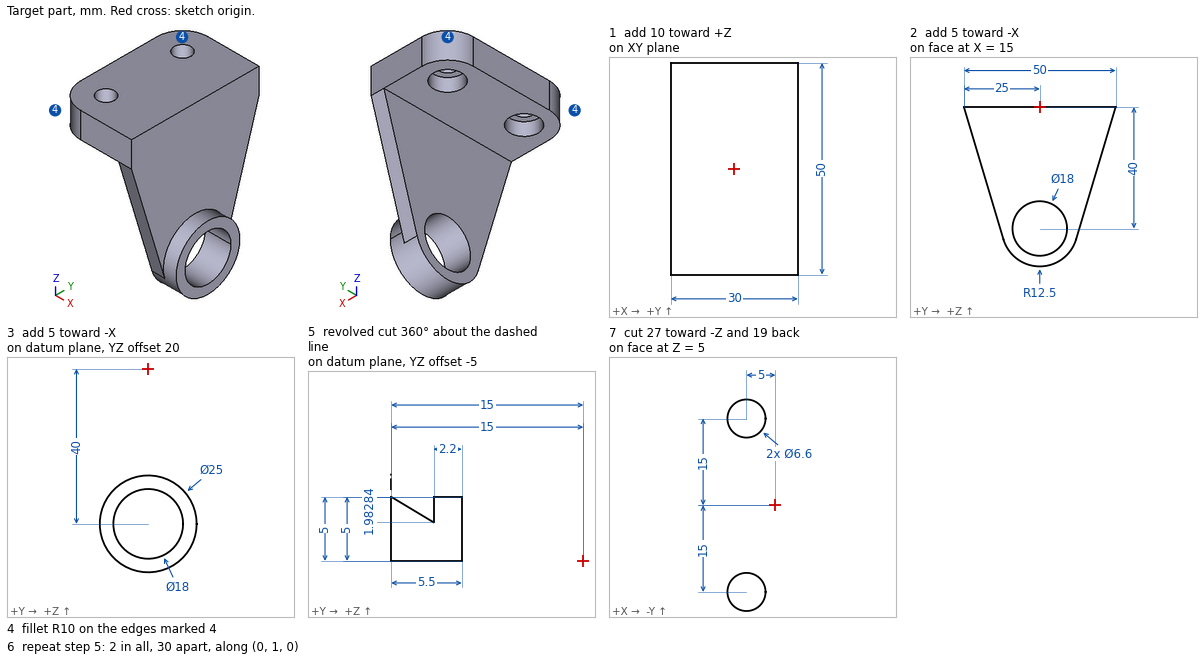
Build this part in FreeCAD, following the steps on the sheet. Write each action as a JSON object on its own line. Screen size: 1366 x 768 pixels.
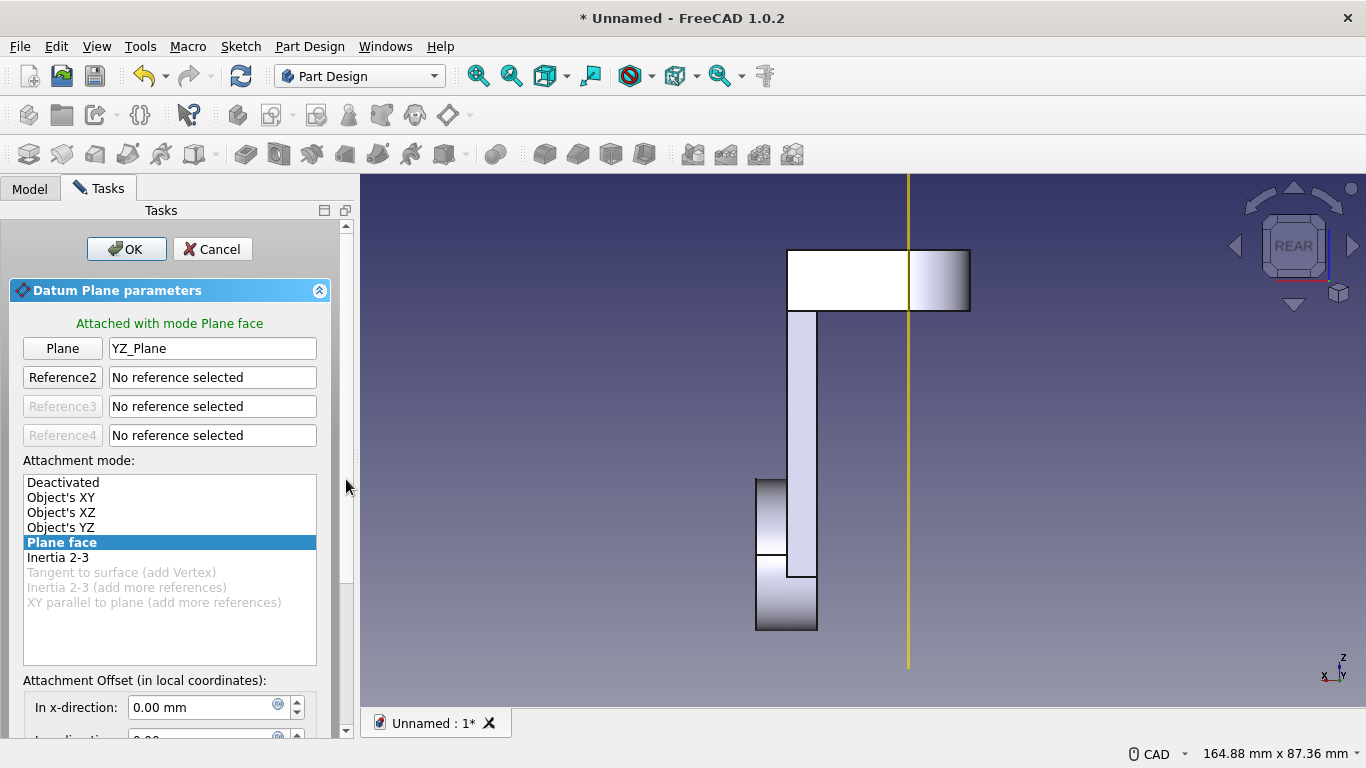
{"action": "left_click", "coordinate": [127, 249]}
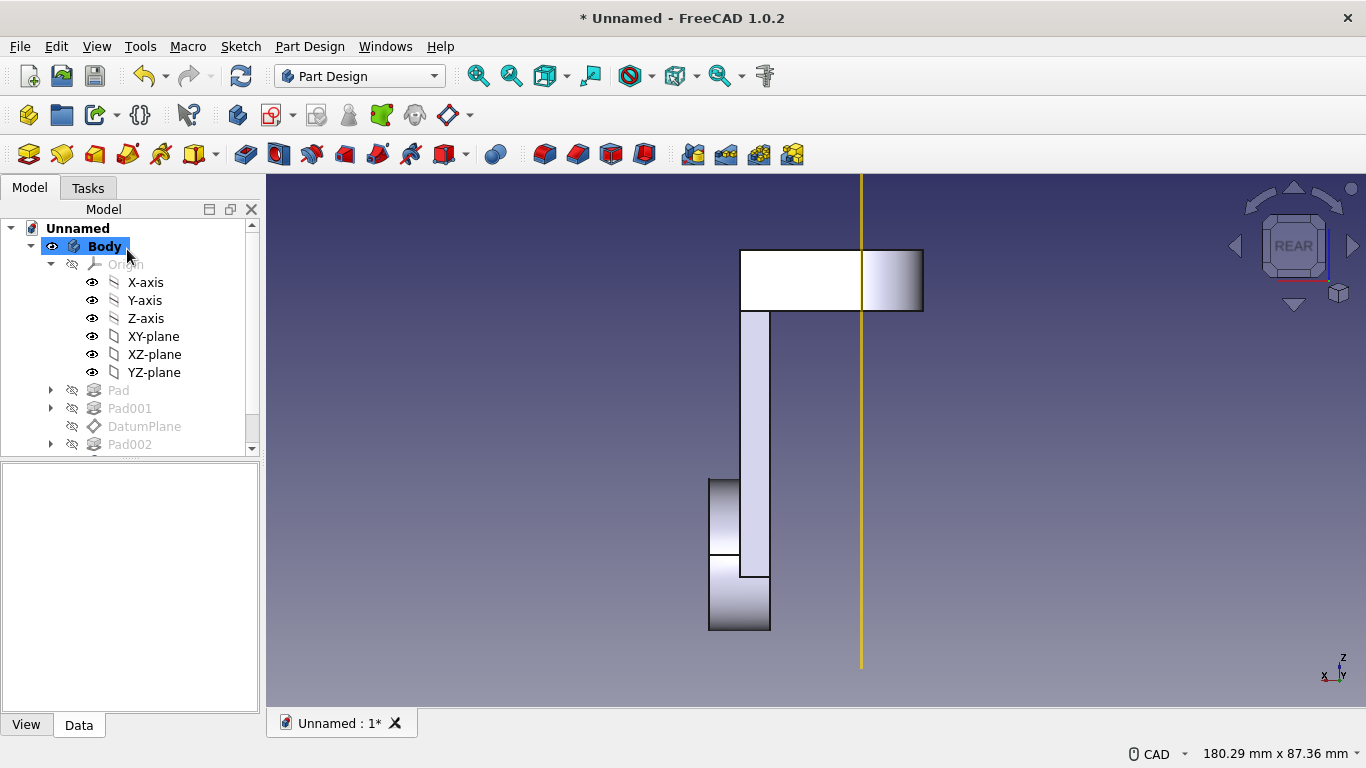
{"action": "scroll", "coordinate": [101, 332], "scroll_direction": "down", "scroll_amount": 3}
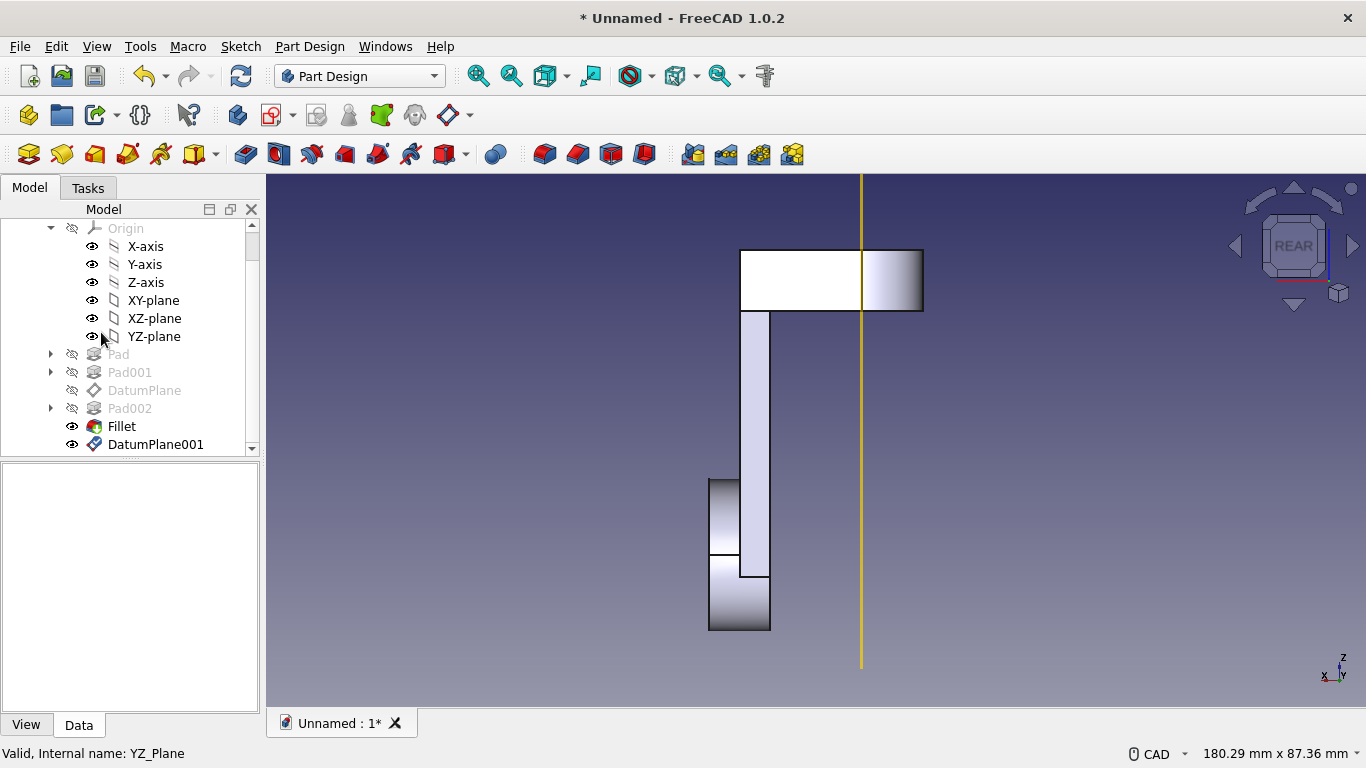
{"action": "left_click", "coordinate": [117, 444]}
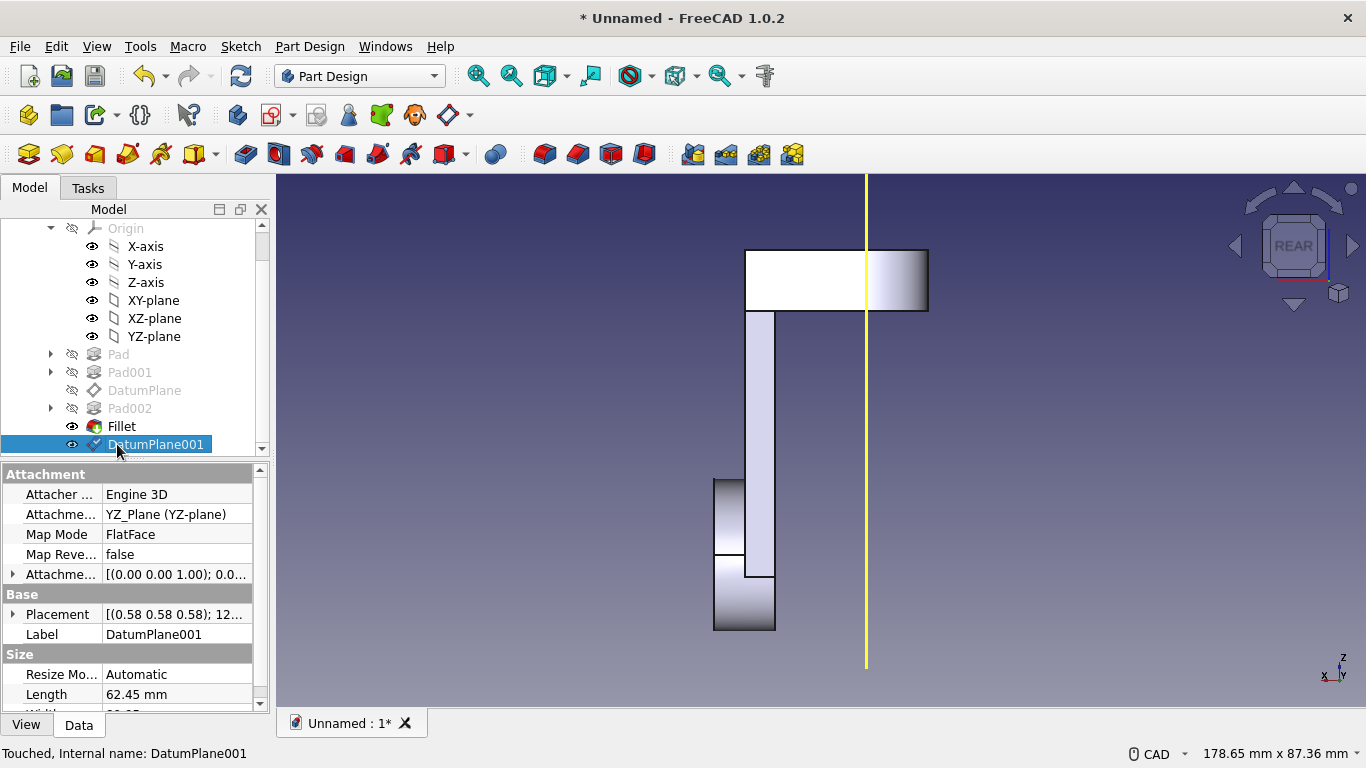
{"action": "left_click", "coordinate": [270, 116]}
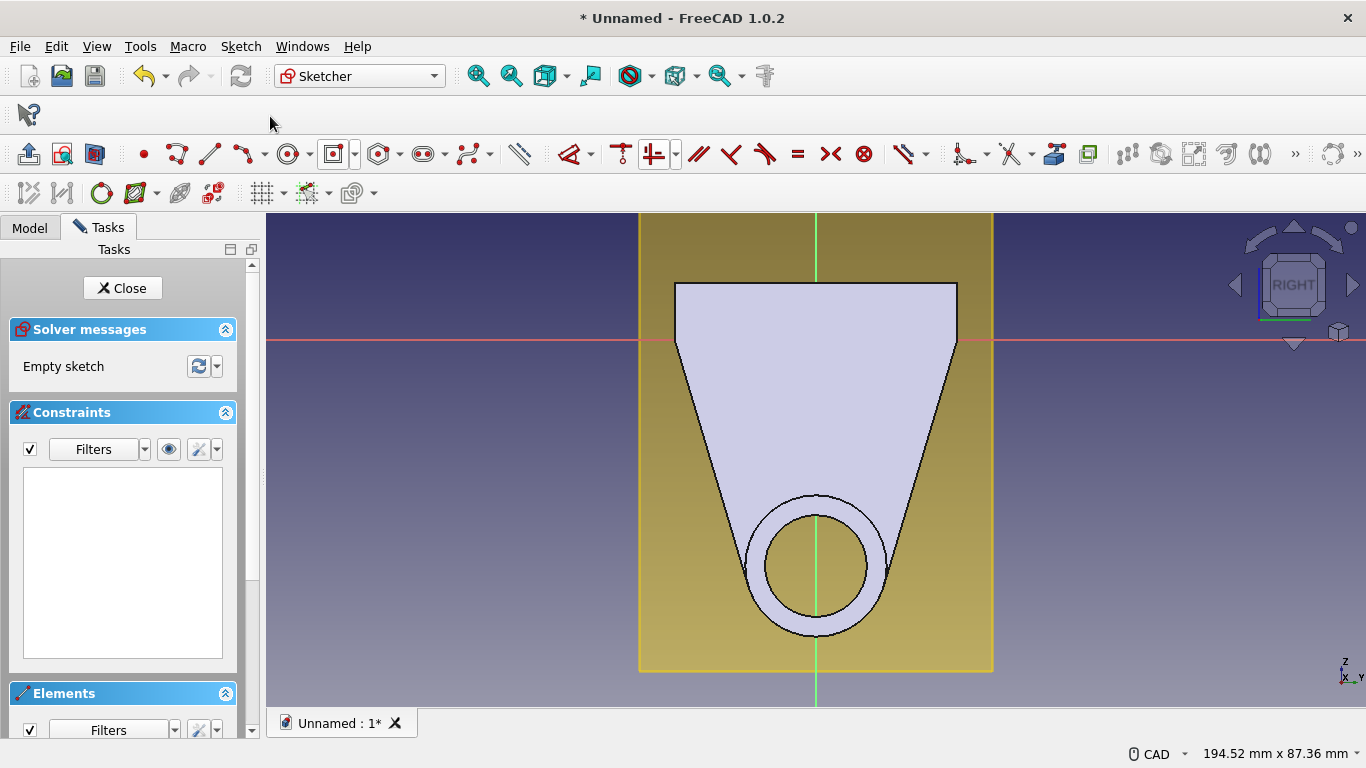
{"action": "left_click", "coordinate": [95, 154]}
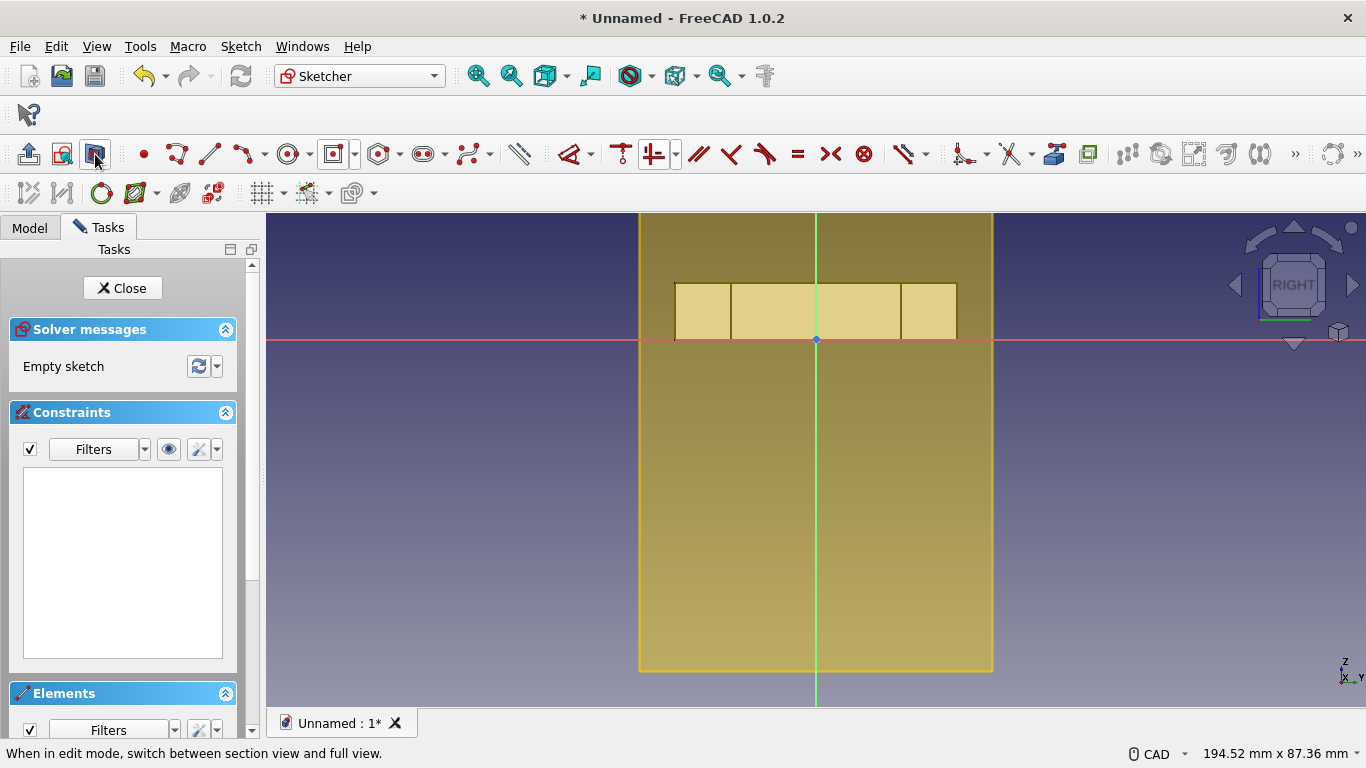
{"action": "scroll", "coordinate": [778, 298], "scroll_direction": "up", "scroll_amount": 10}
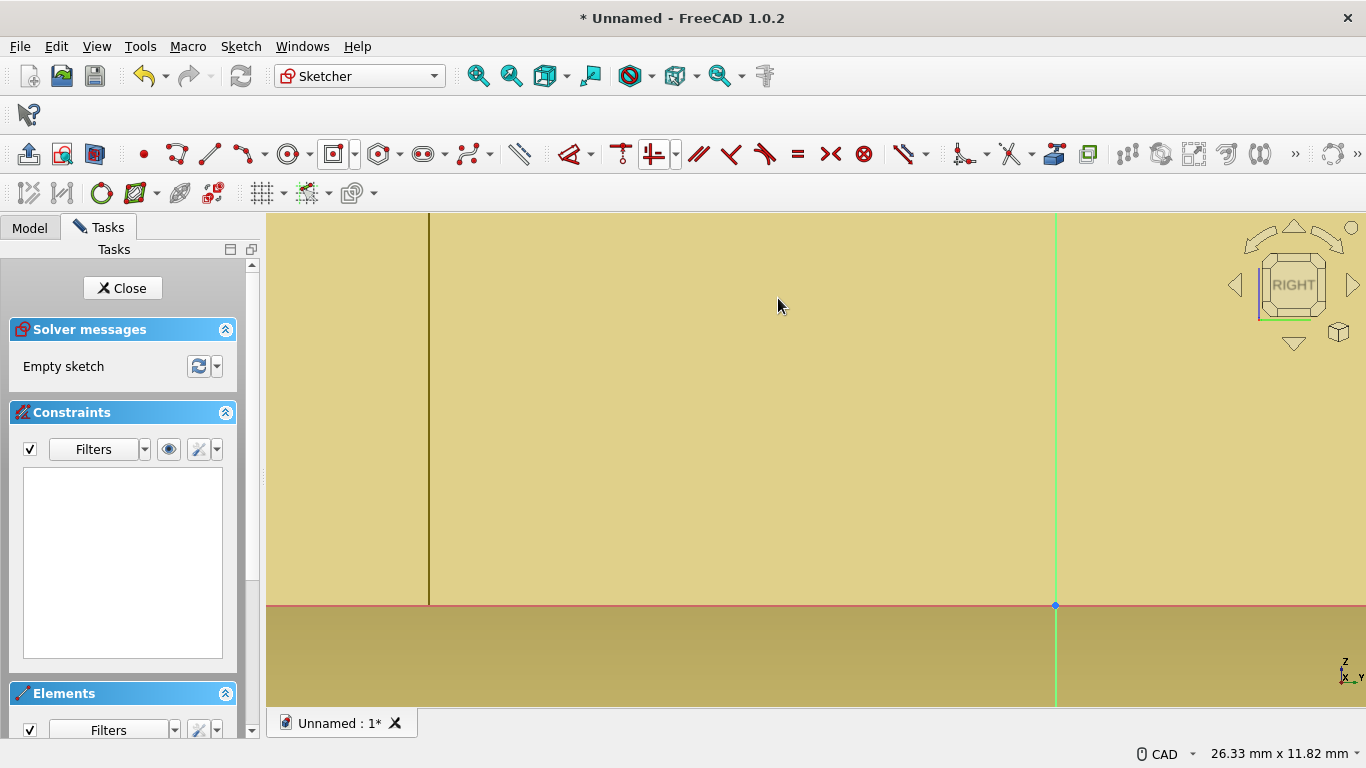
{"action": "left_click", "coordinate": [177, 154]}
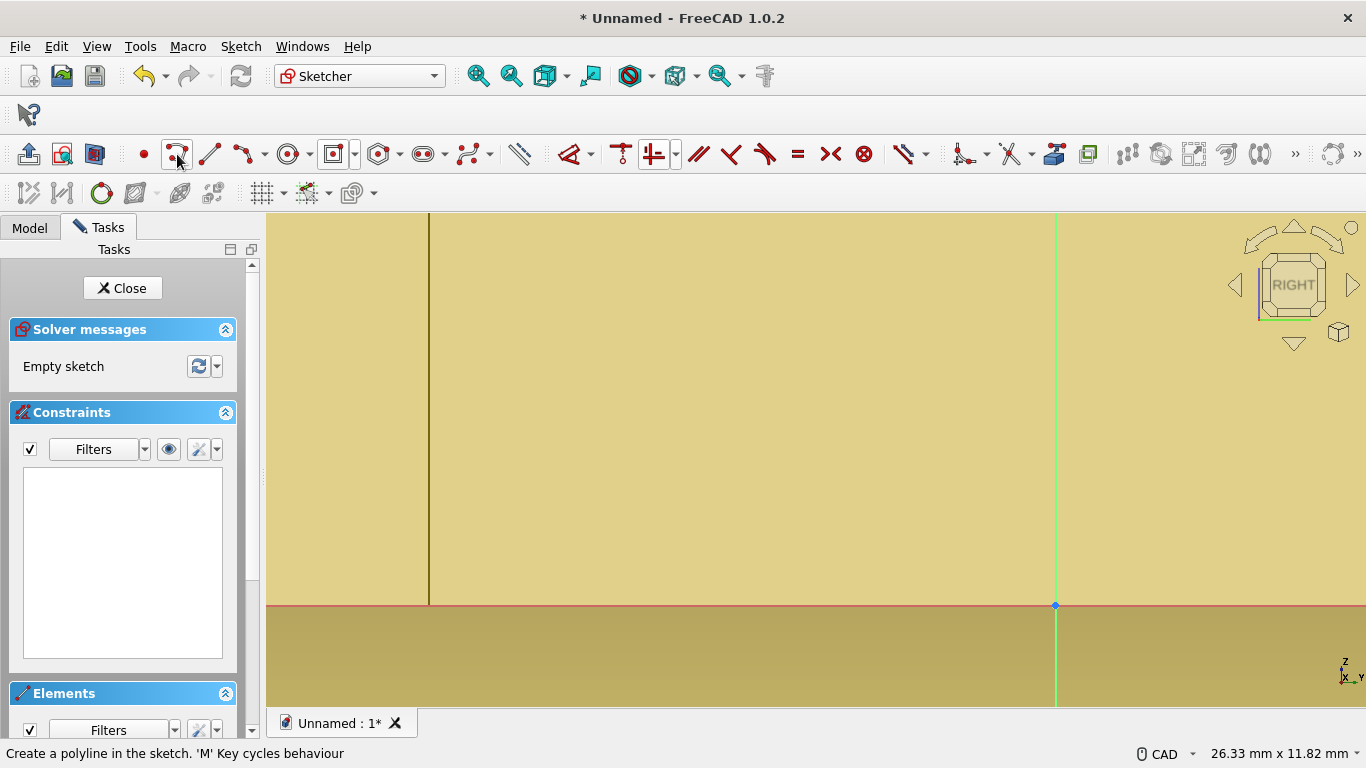
{"action": "left_click", "coordinate": [659, 606]}
{"action": "left_click", "coordinate": [659, 397]}
{"action": "left_click", "coordinate": [567, 397]}
{"action": "left_click", "coordinate": [567, 480]}
{"action": "left_click", "coordinate": [429, 397]}
{"action": "left_click", "coordinate": [429, 597]}
{"action": "left_click", "coordinate": [659, 606]}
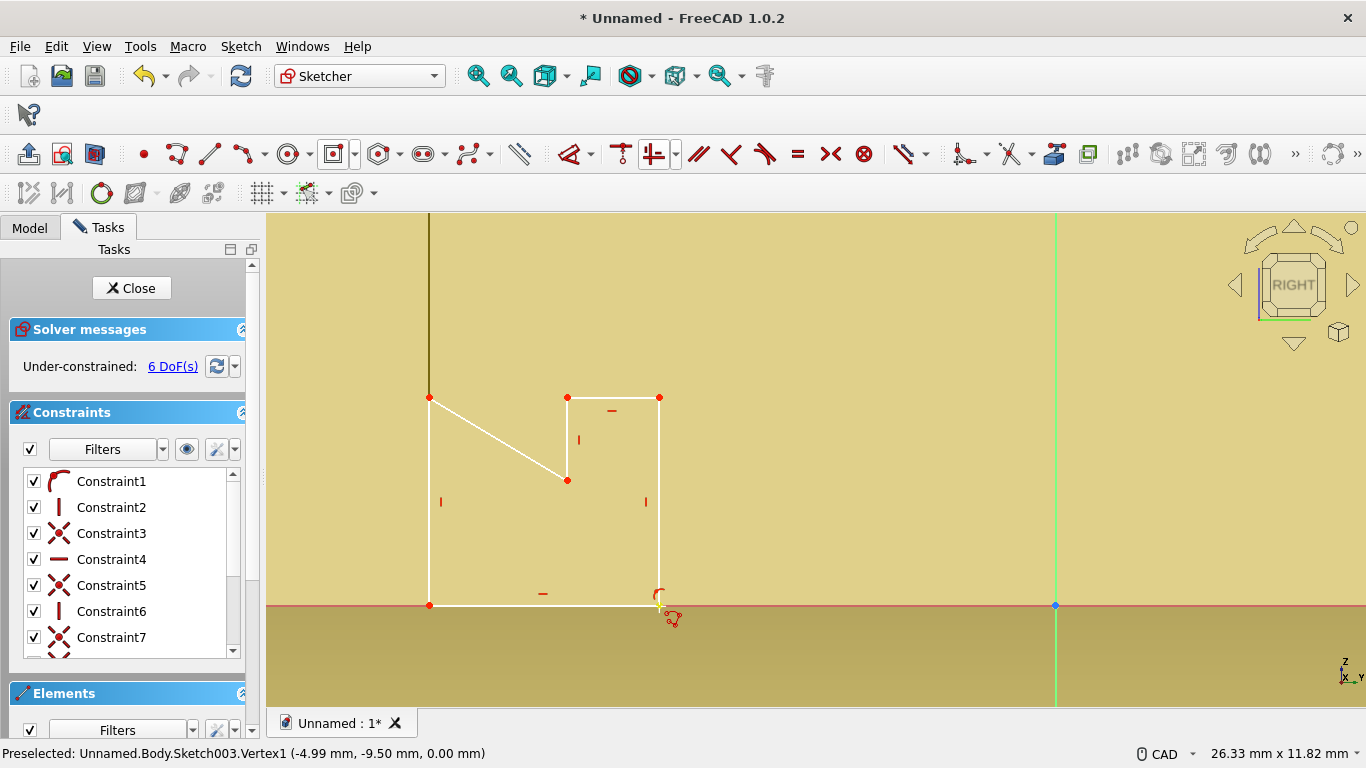
{"action": "key", "text": "g l"}